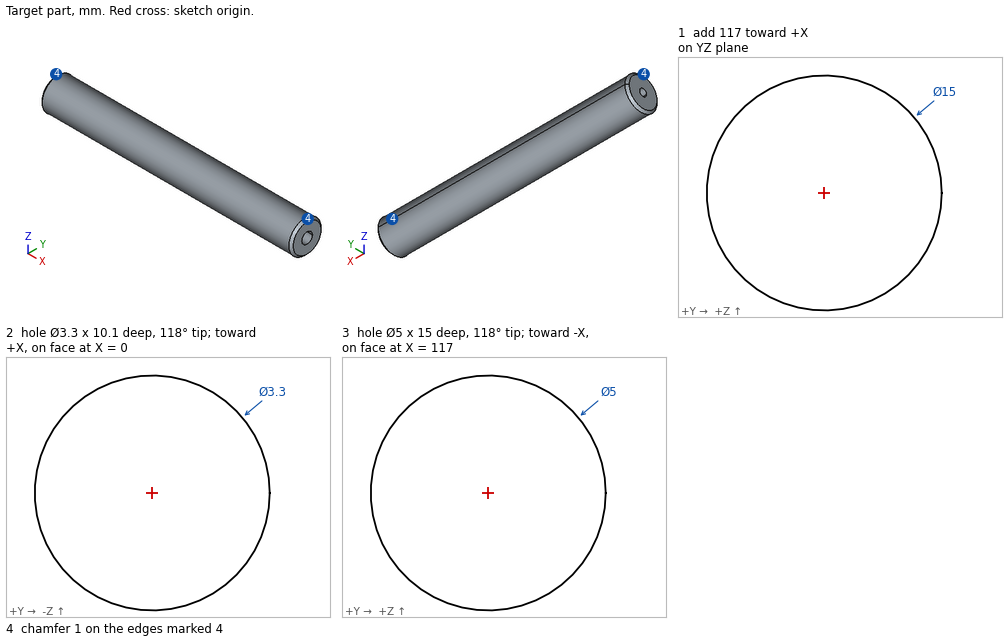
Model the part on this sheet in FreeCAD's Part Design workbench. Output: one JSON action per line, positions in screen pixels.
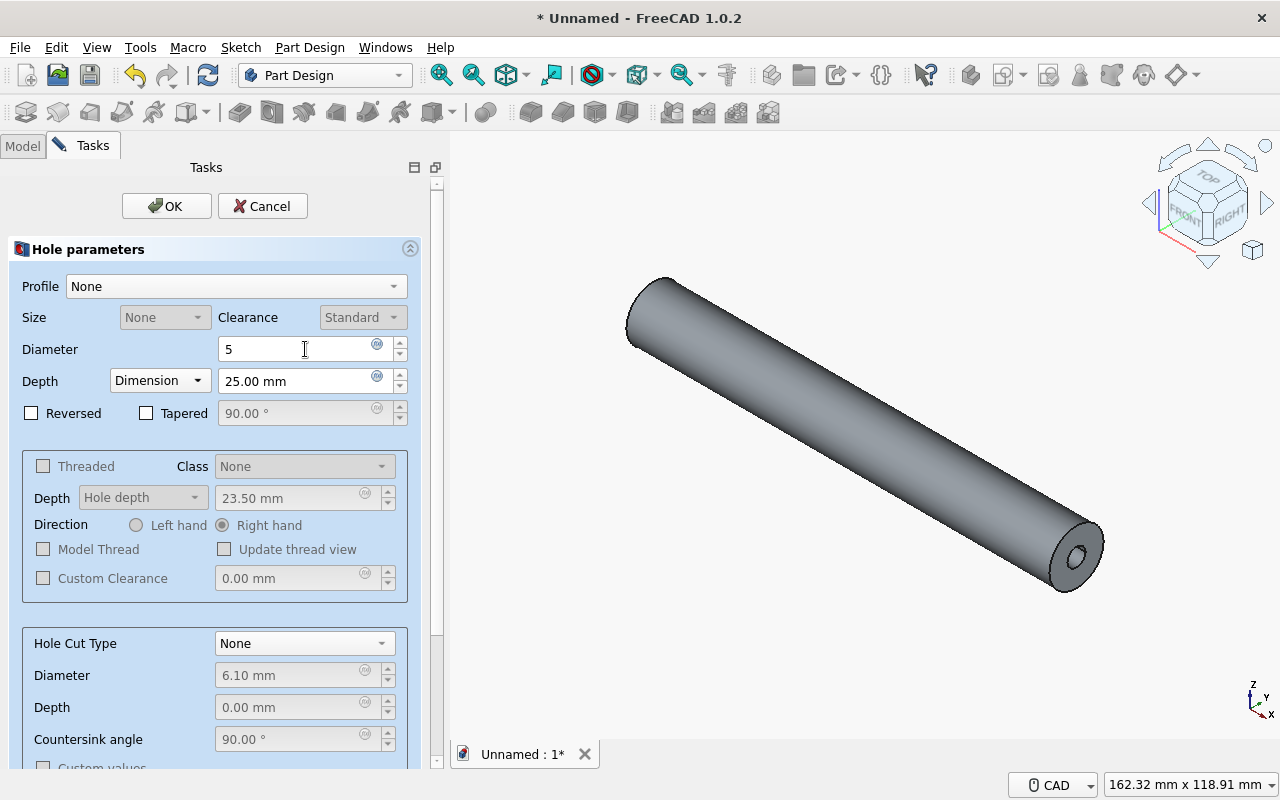
{"action": "triple_click", "coordinate": [305, 381]}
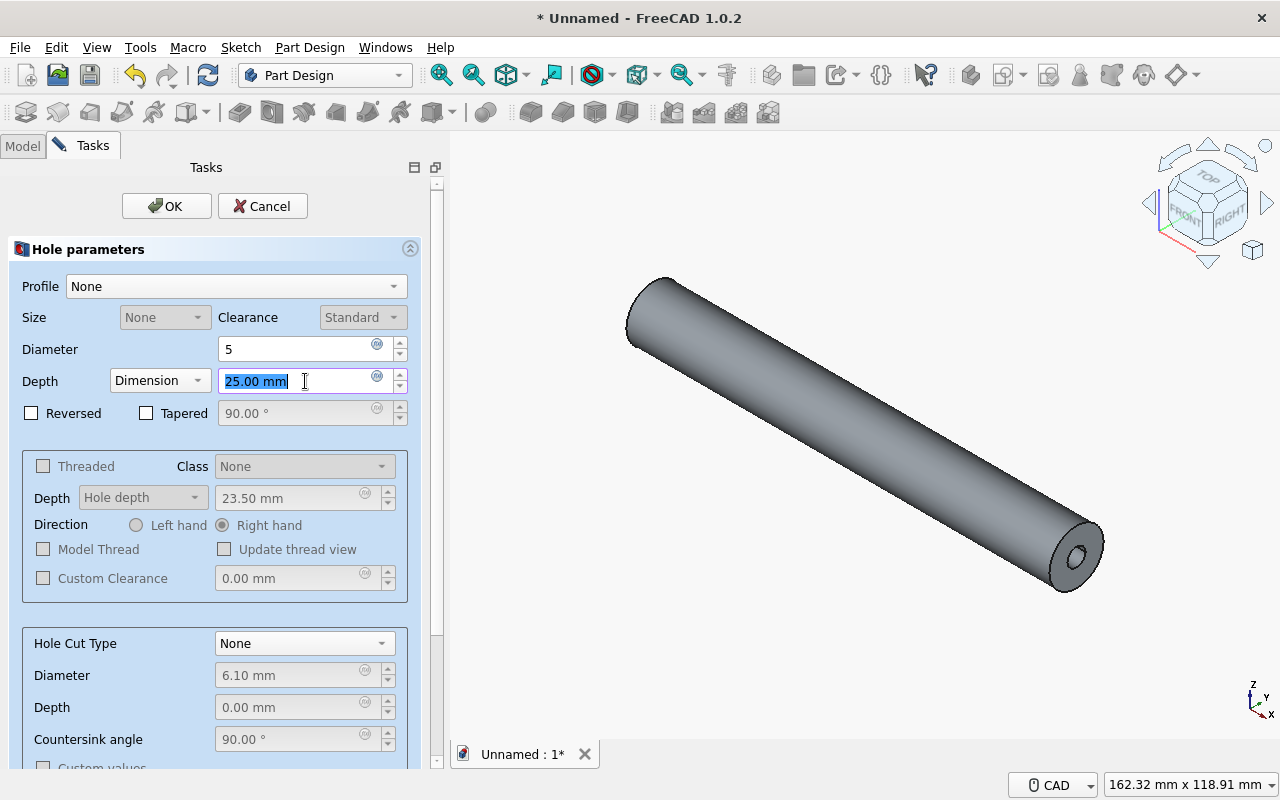
{"action": "type", "text": "15"}
{"action": "key", "text": "Tab"}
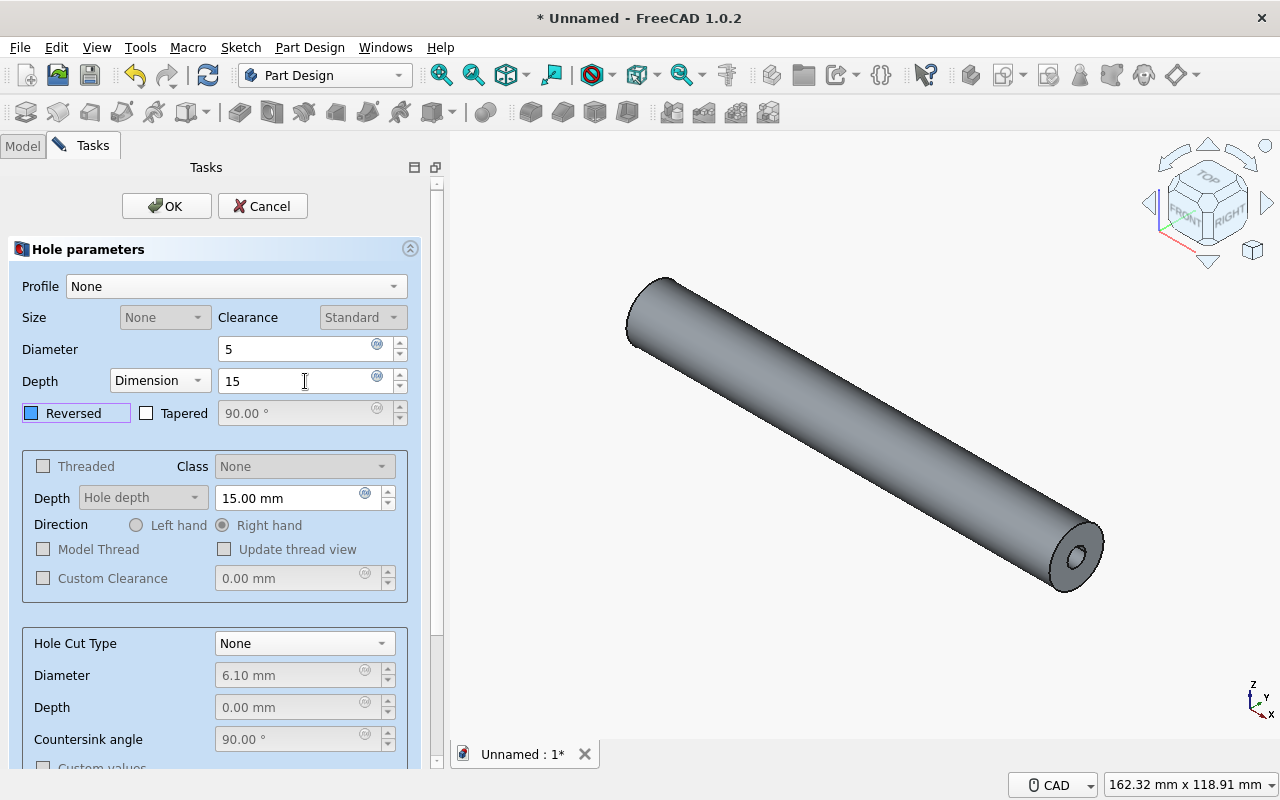
{"action": "left_click", "coordinate": [167, 206]}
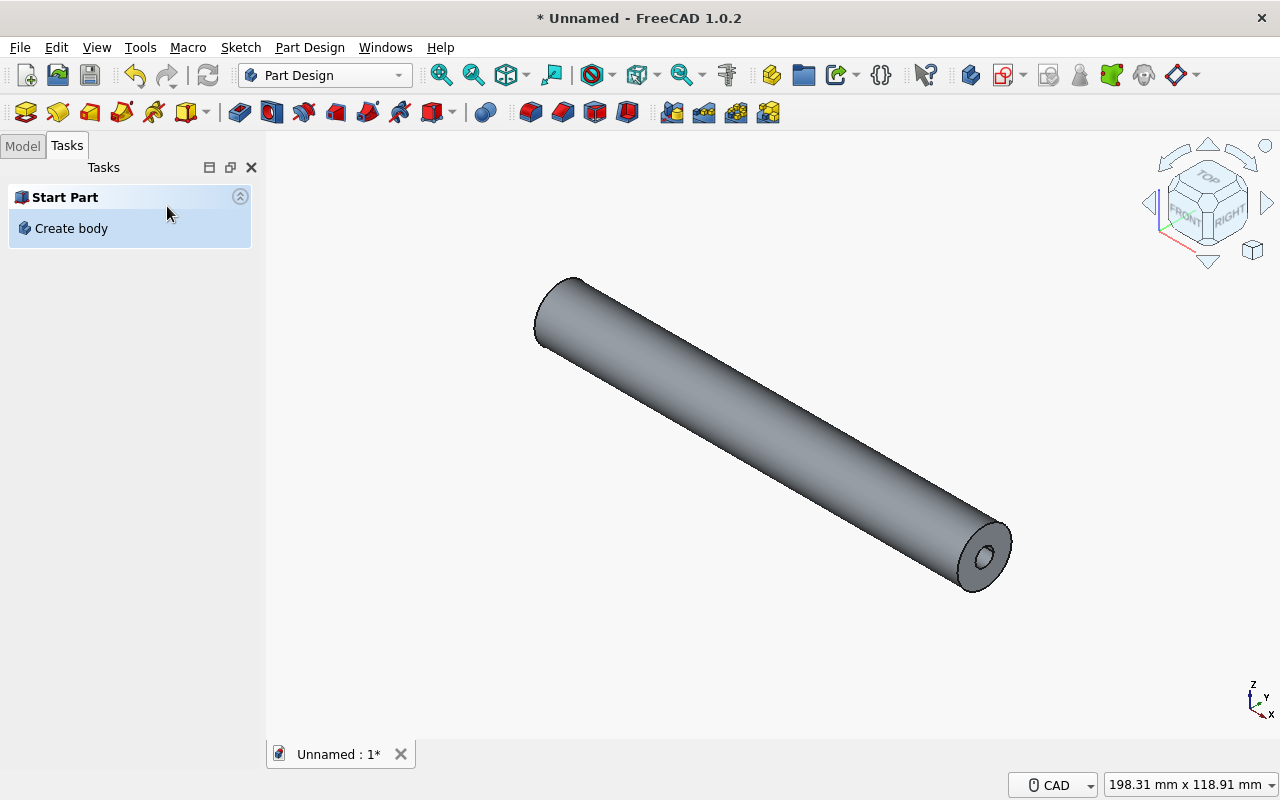
{"action": "left_click", "coordinate": [570, 277]}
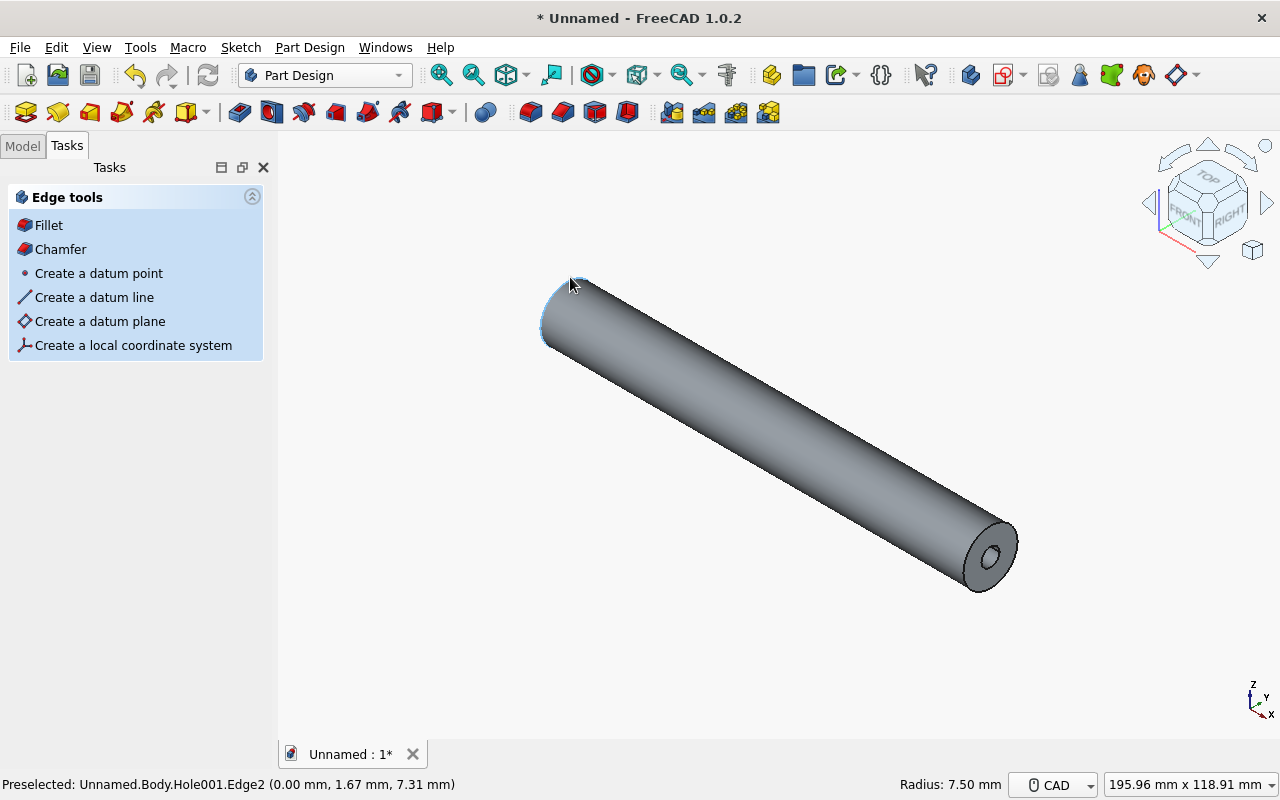
{"action": "left_click", "coordinate": [963, 572], "text": "ctrl"}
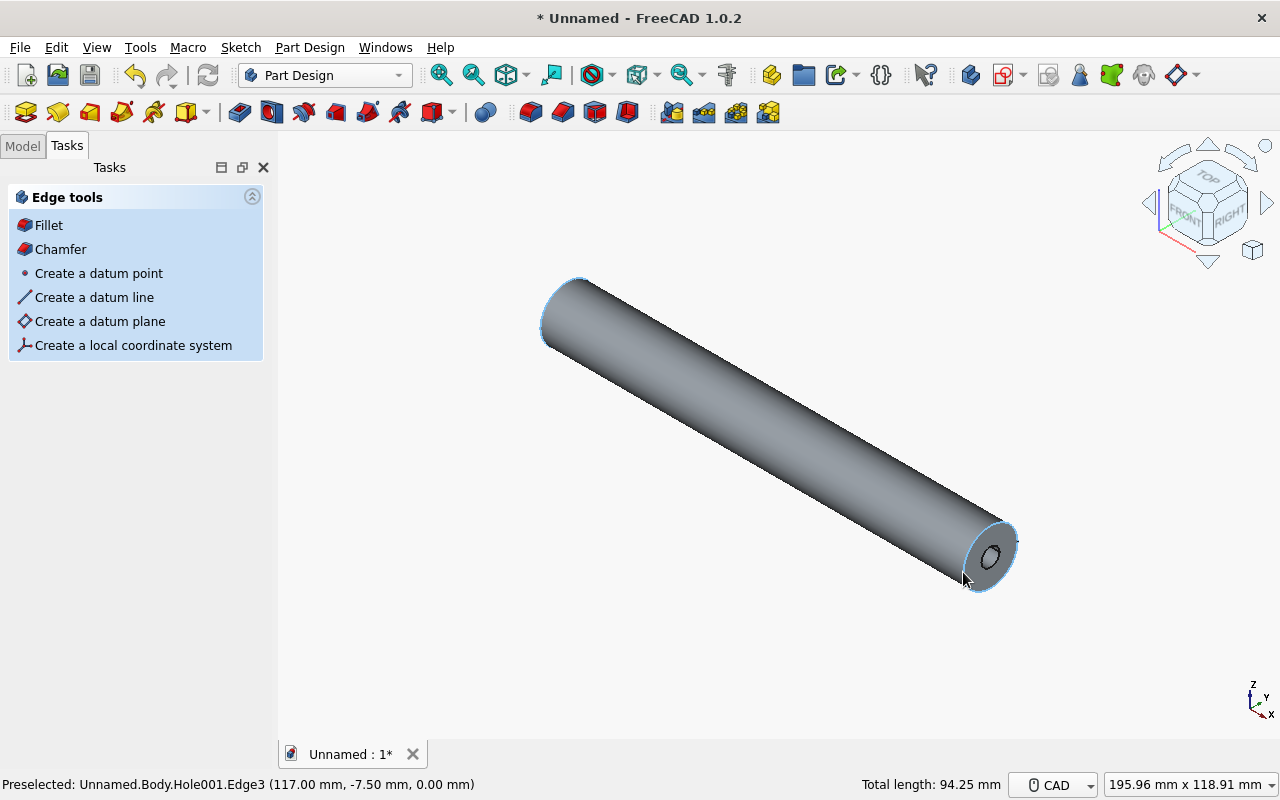
{"action": "left_click", "coordinate": [564, 112]}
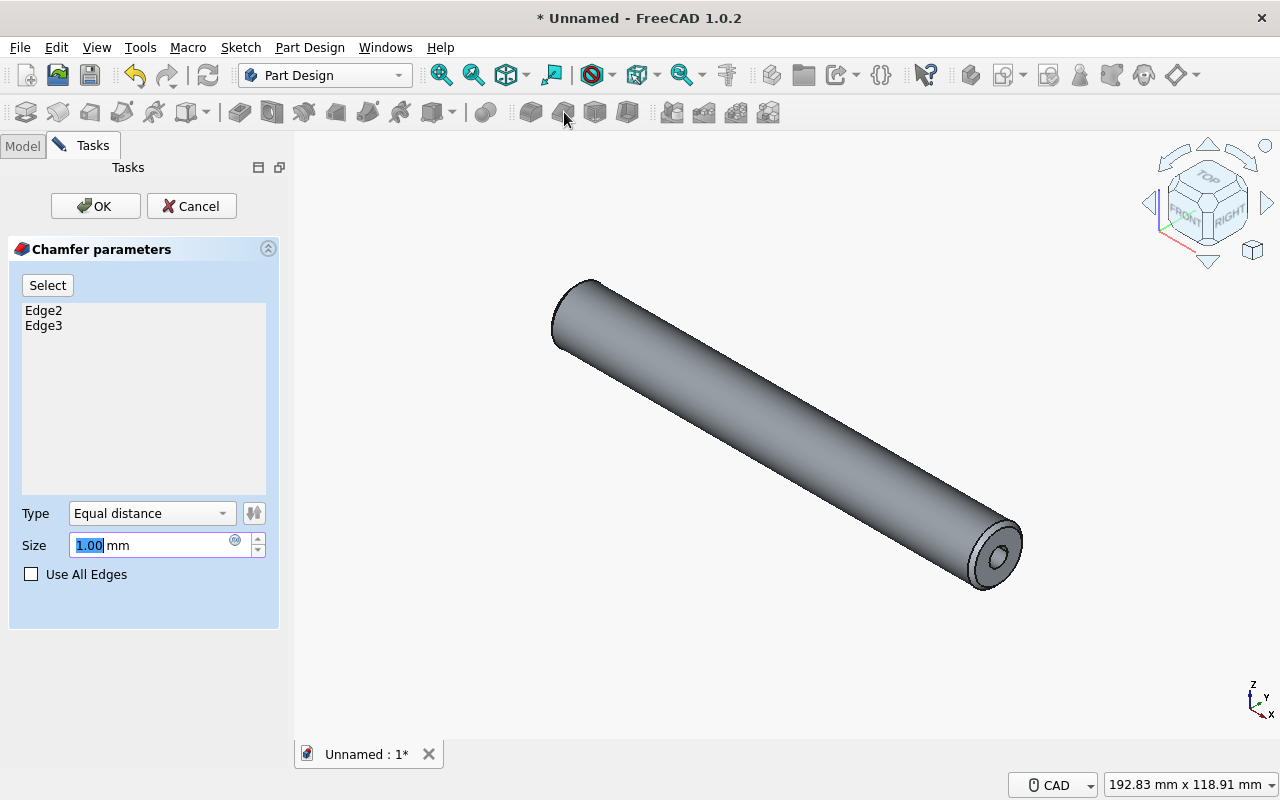
{"action": "type", "text": "1"}
{"action": "key", "text": "Tab"}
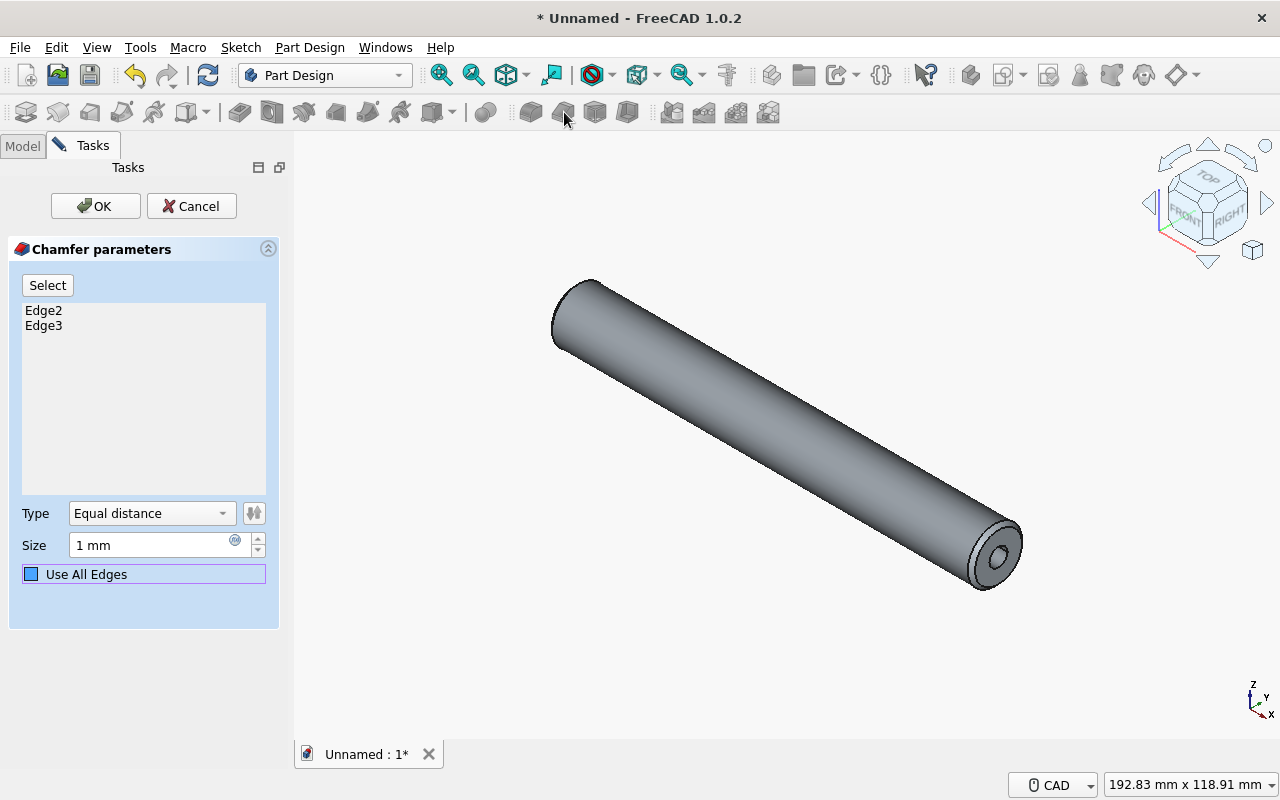
{"action": "left_click", "coordinate": [96, 206]}